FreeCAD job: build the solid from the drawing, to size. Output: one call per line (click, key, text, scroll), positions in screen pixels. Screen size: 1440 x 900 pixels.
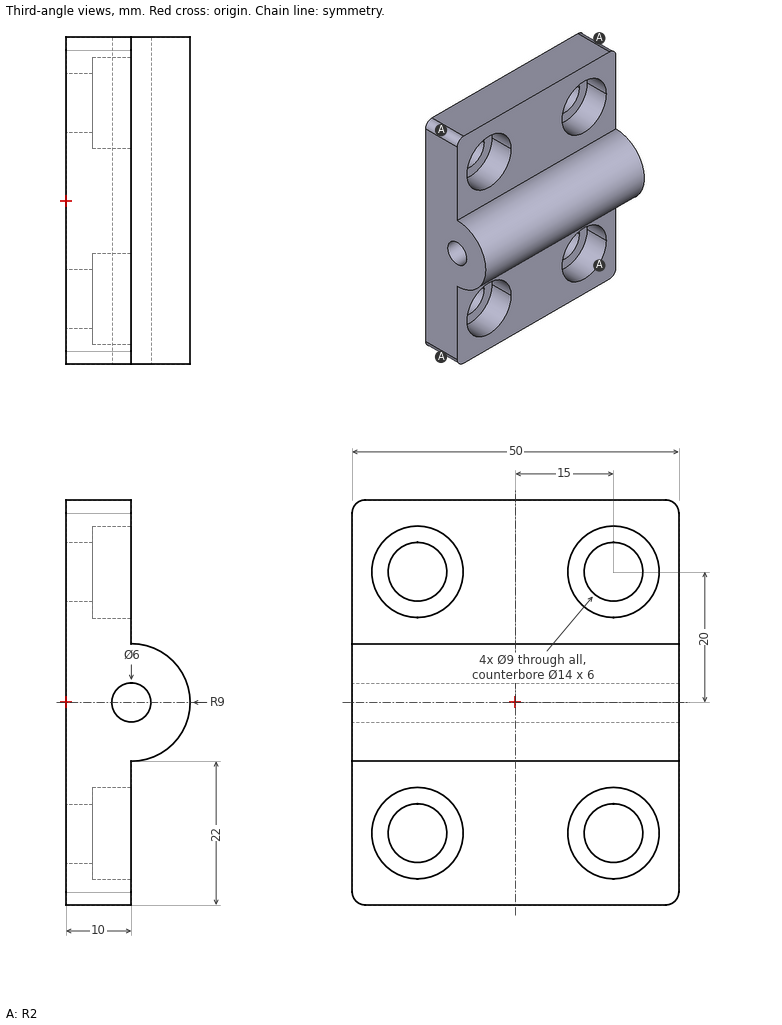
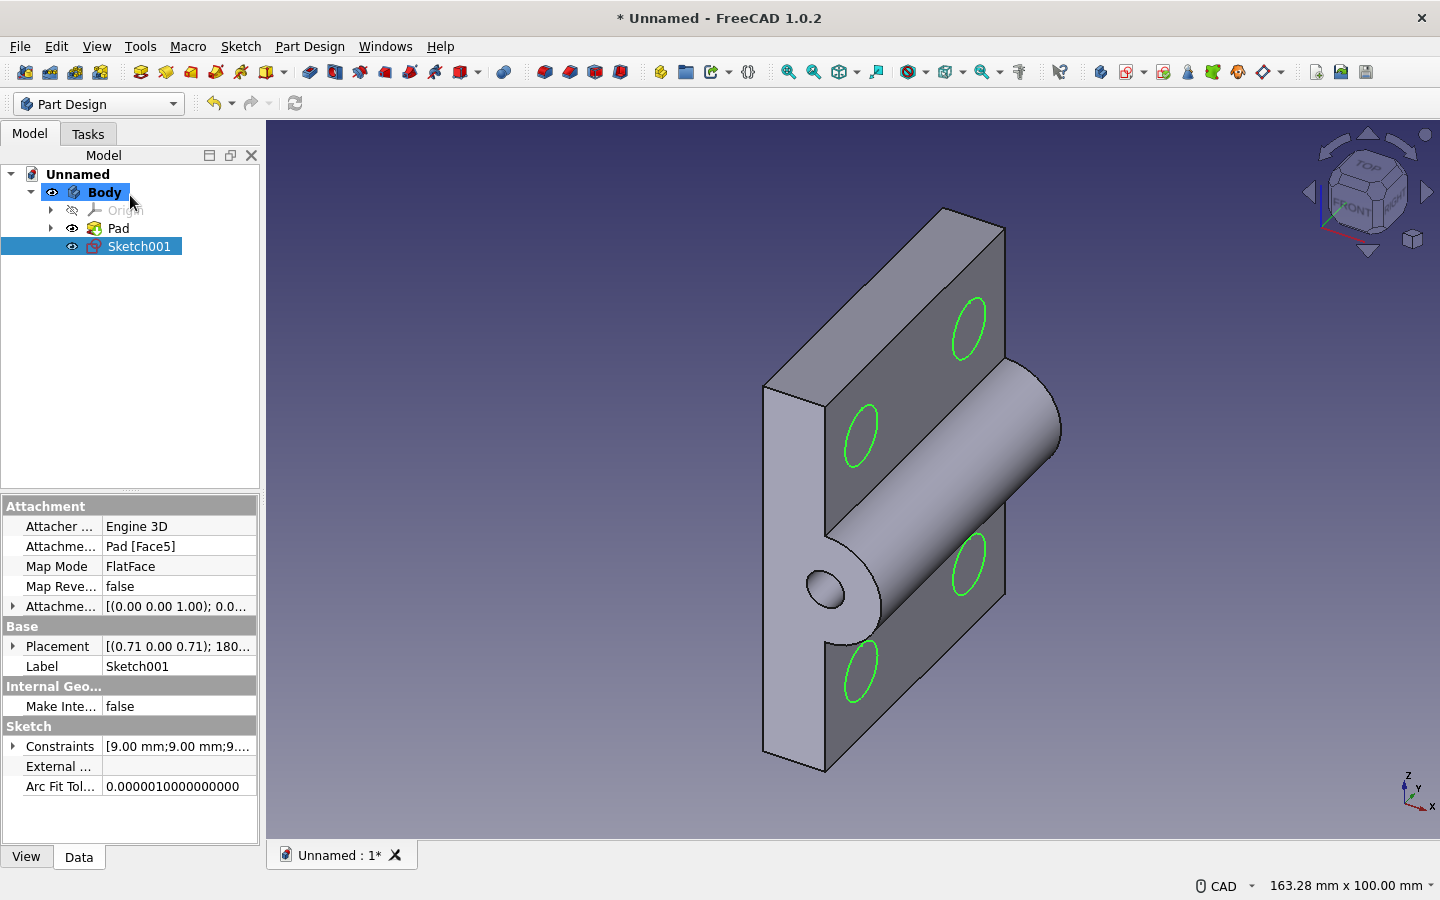
click(335, 72)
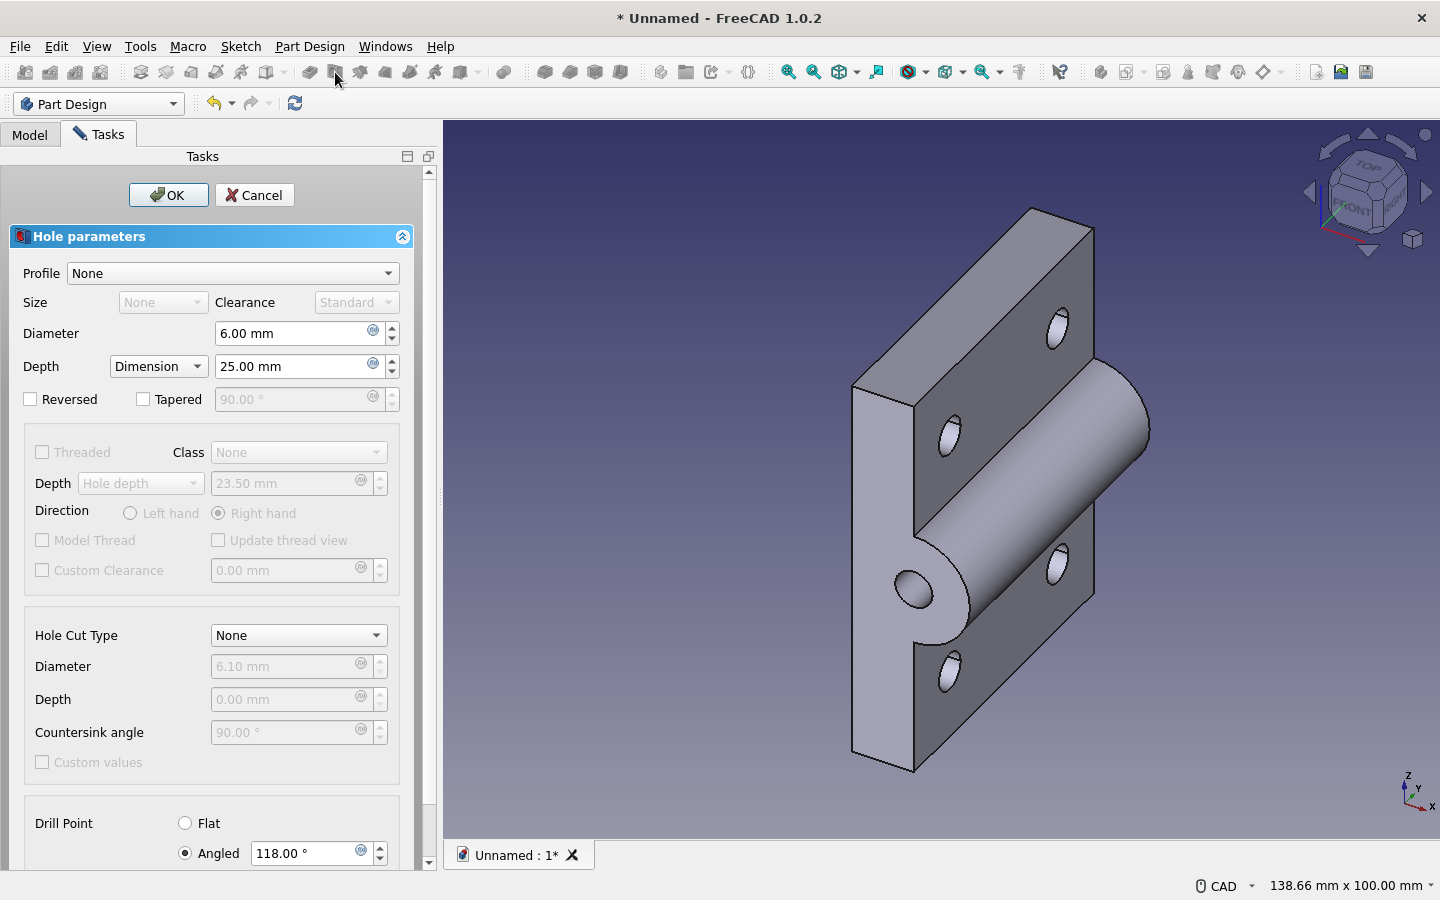
triple_click(300, 334)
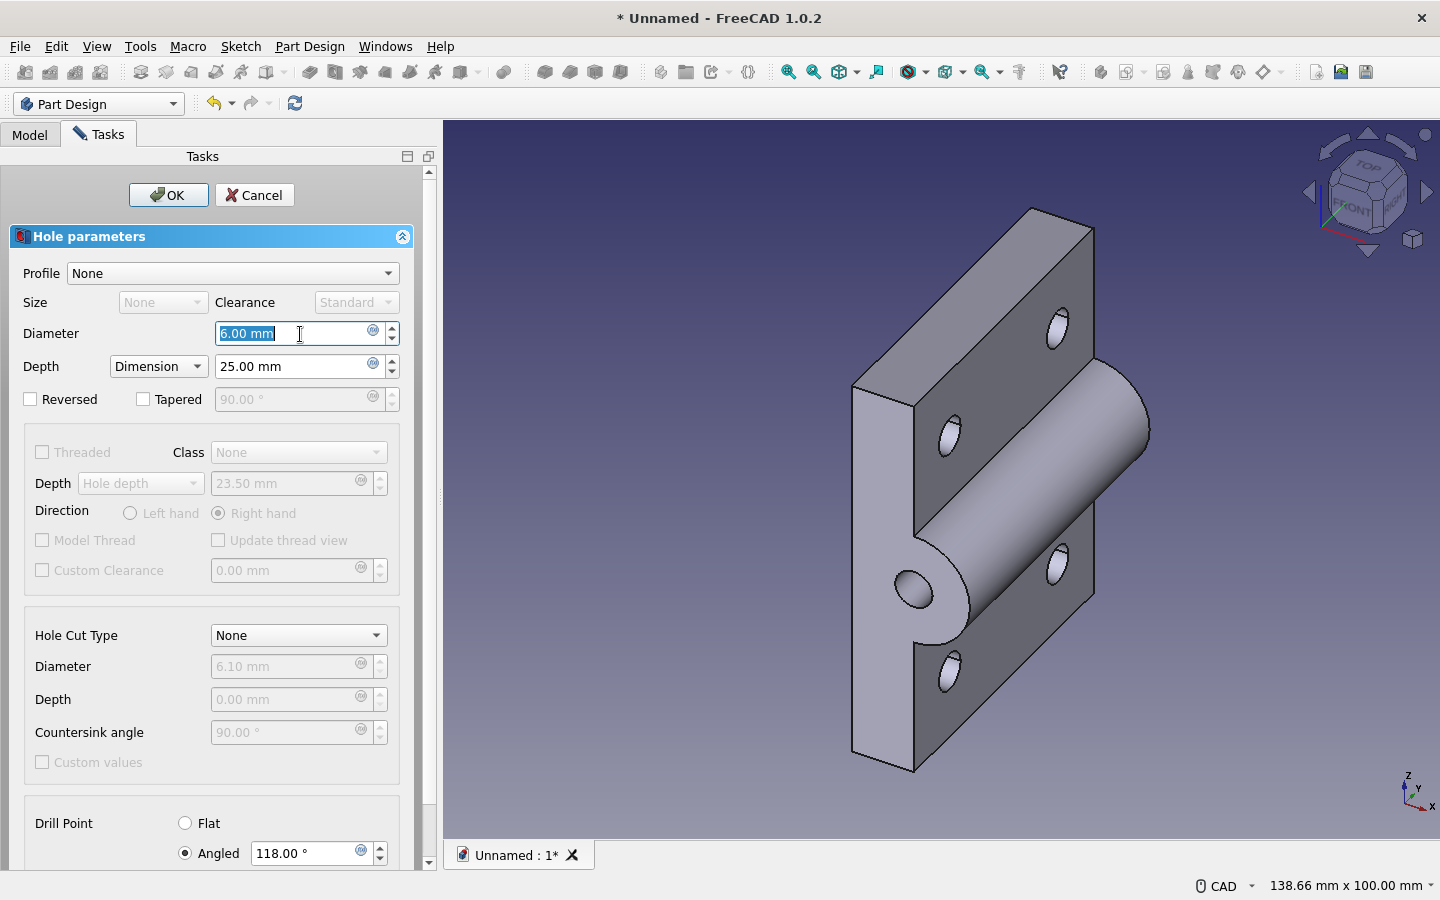
text(9)
key(Tab)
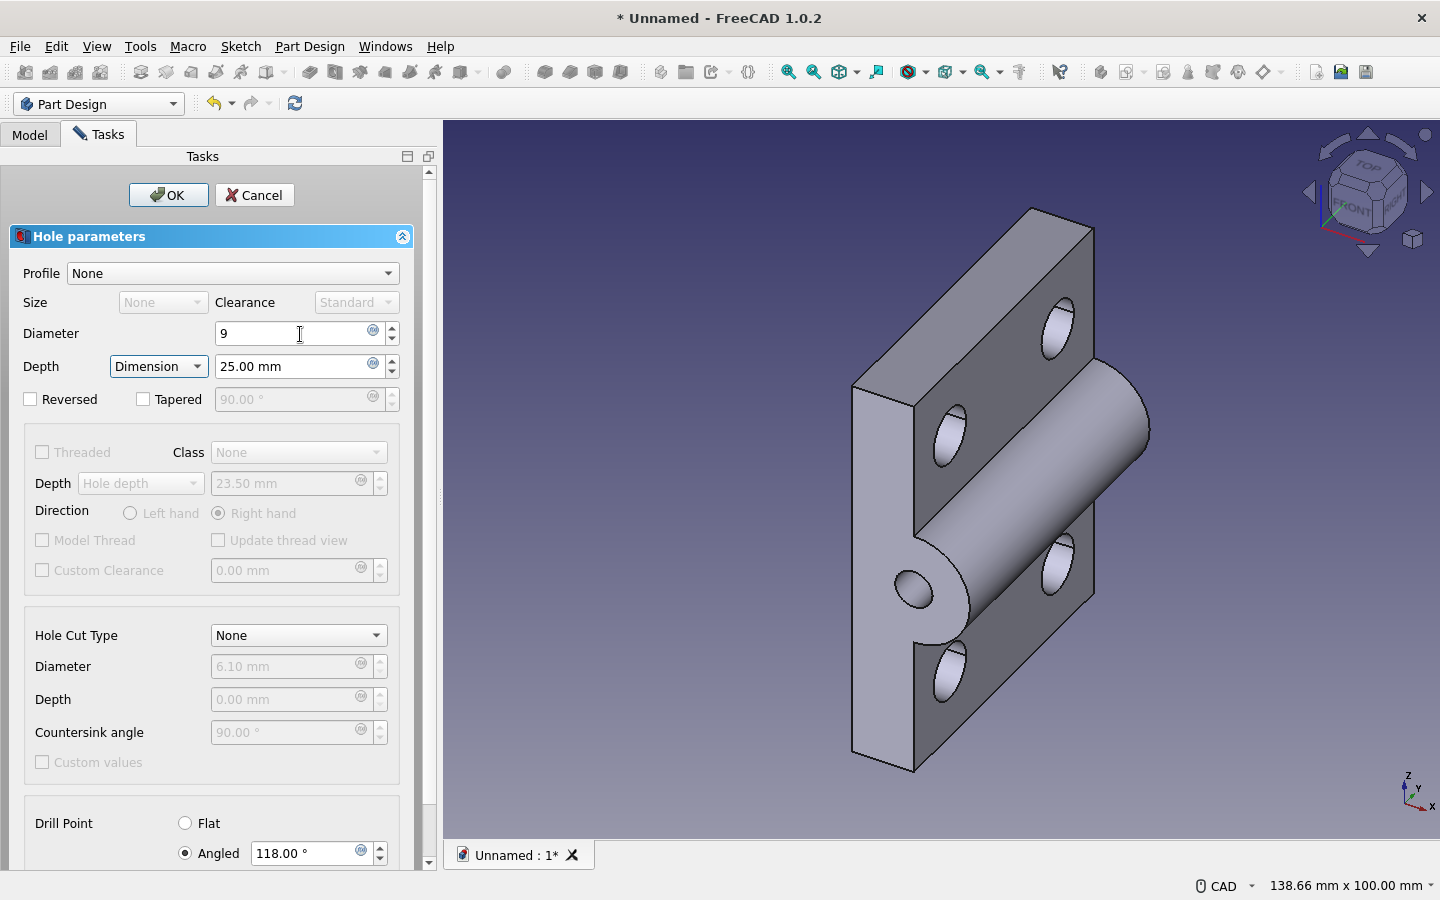
click(160, 366)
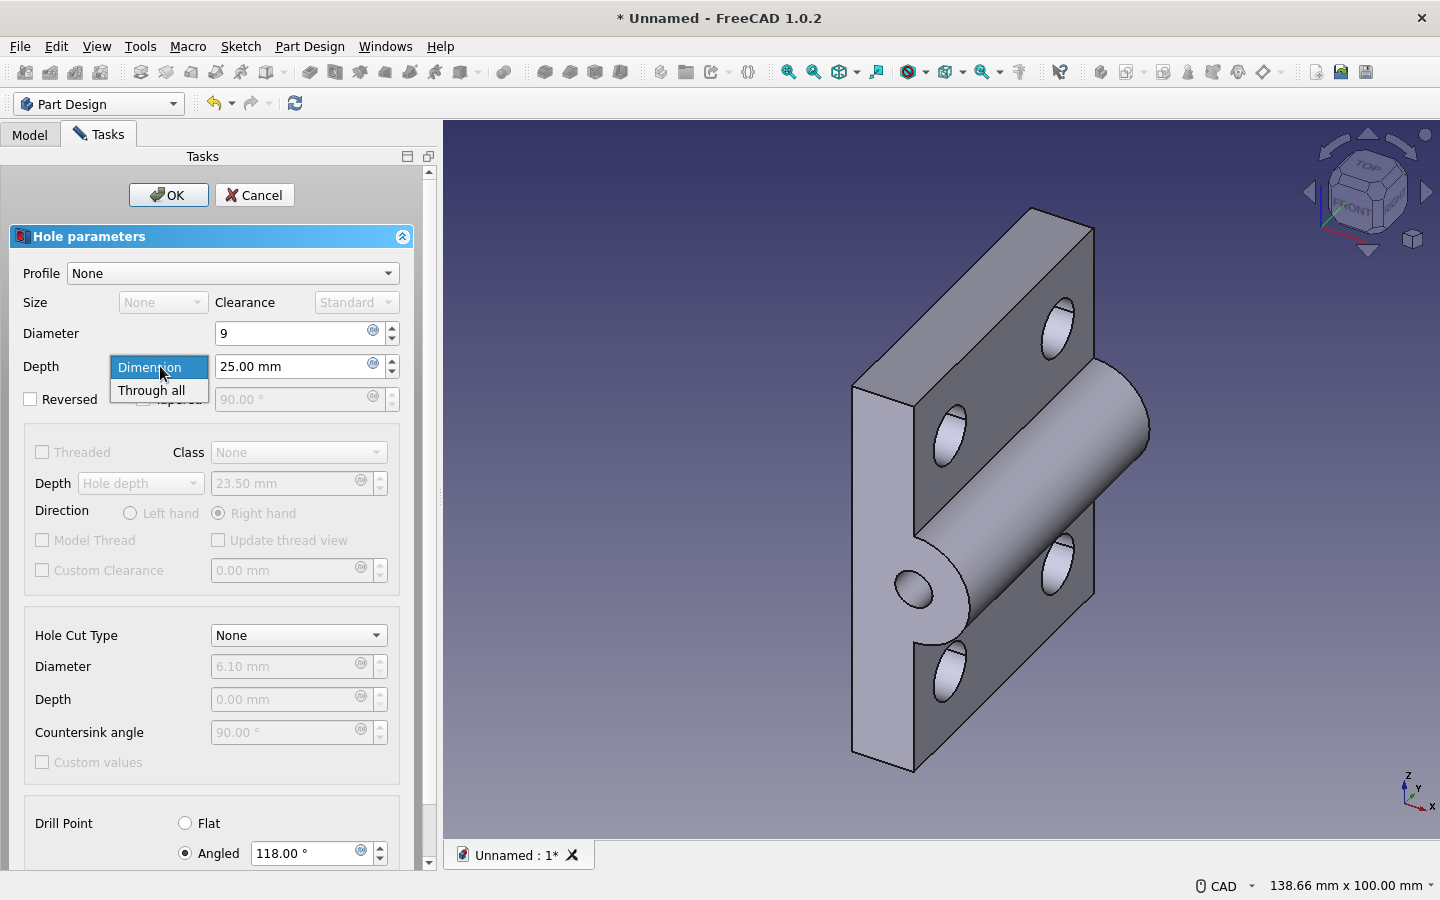
click(158, 390)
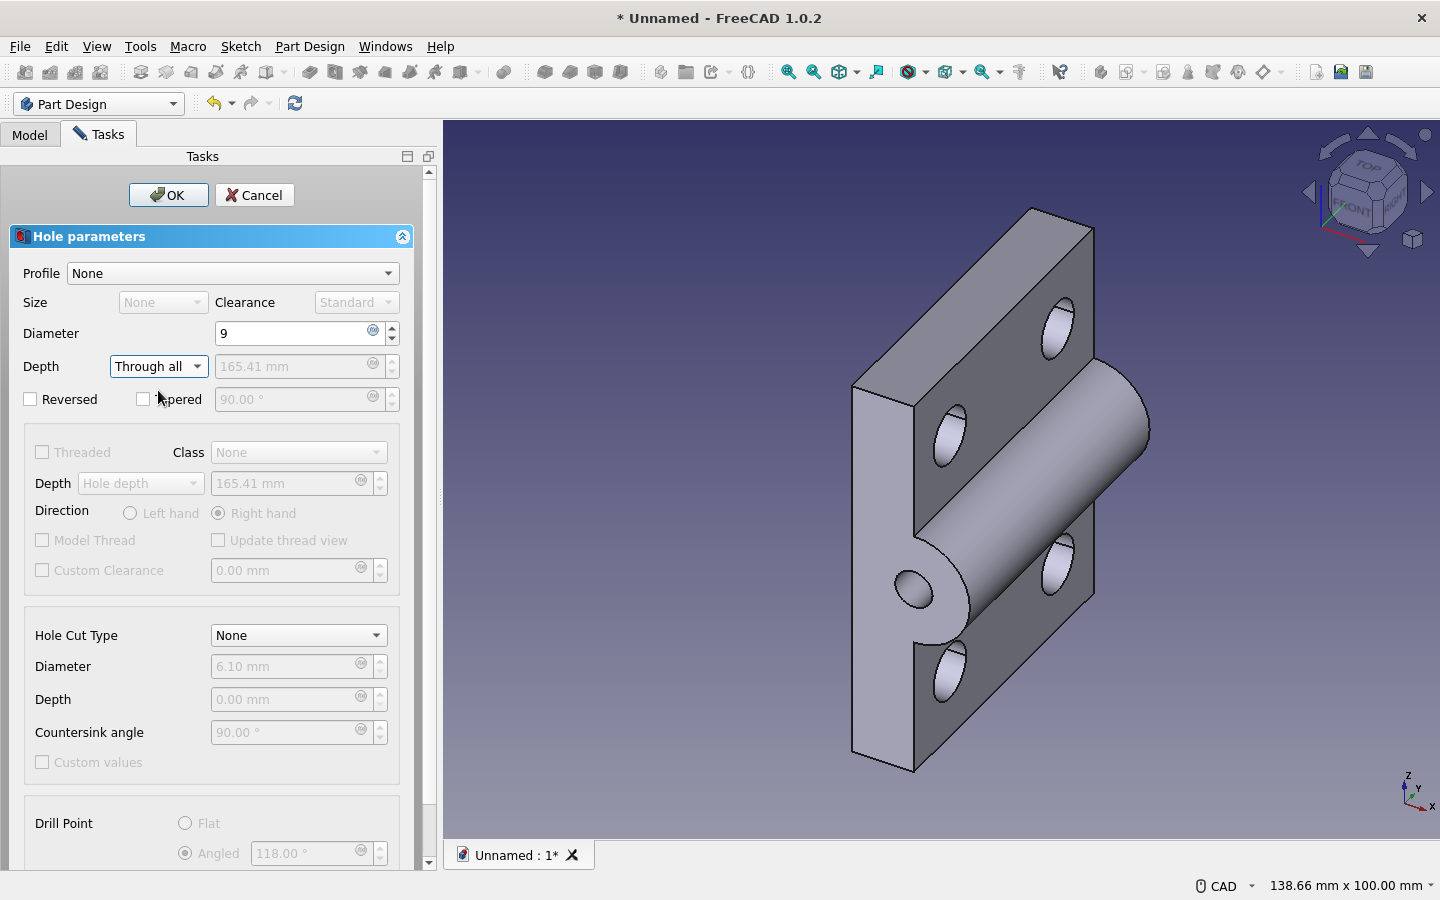
click(300, 636)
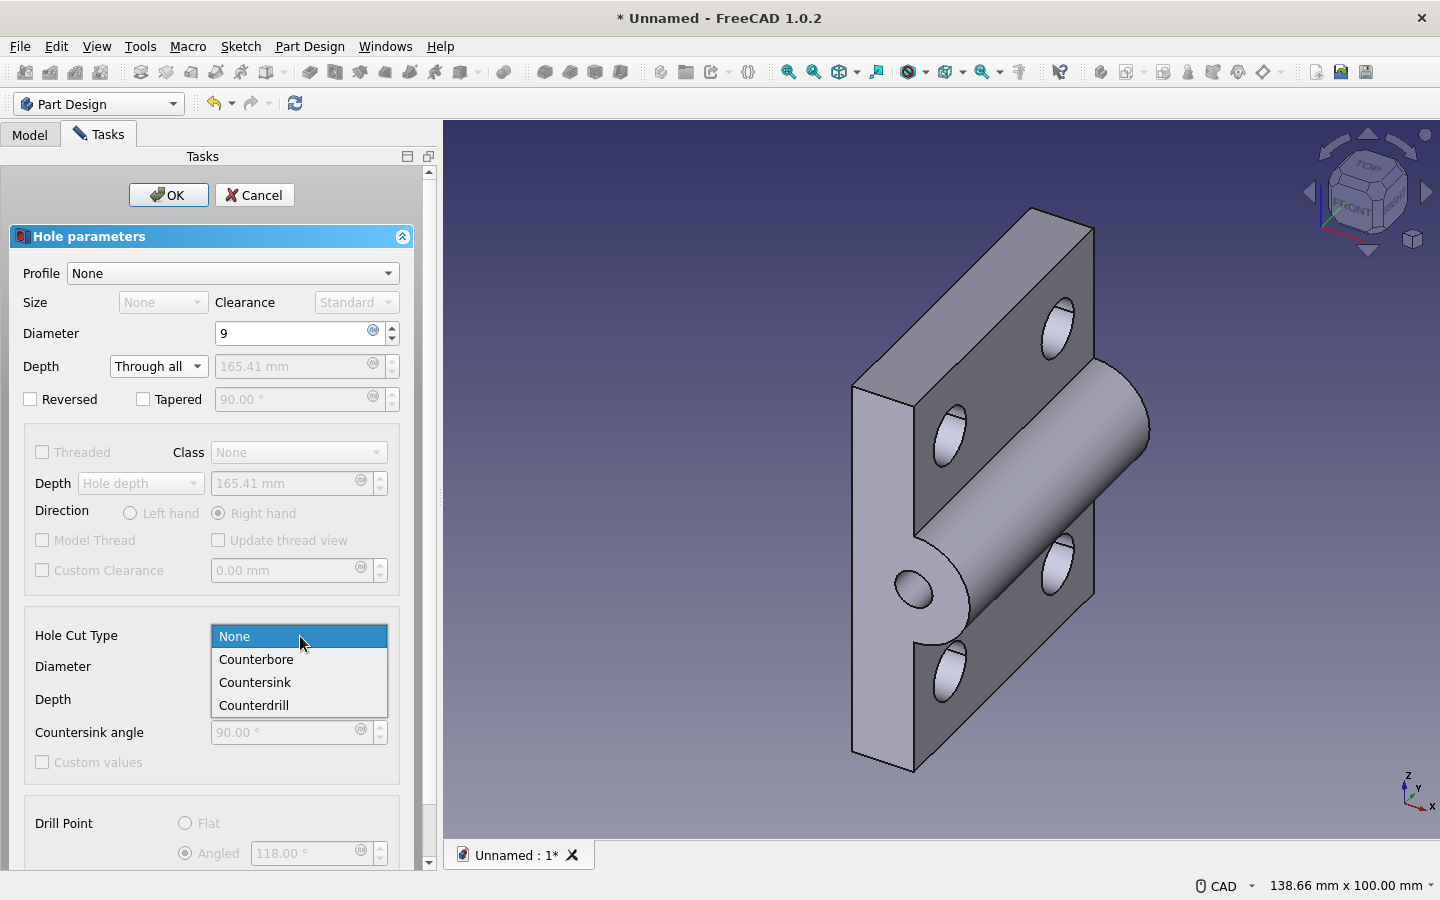
click(298, 660)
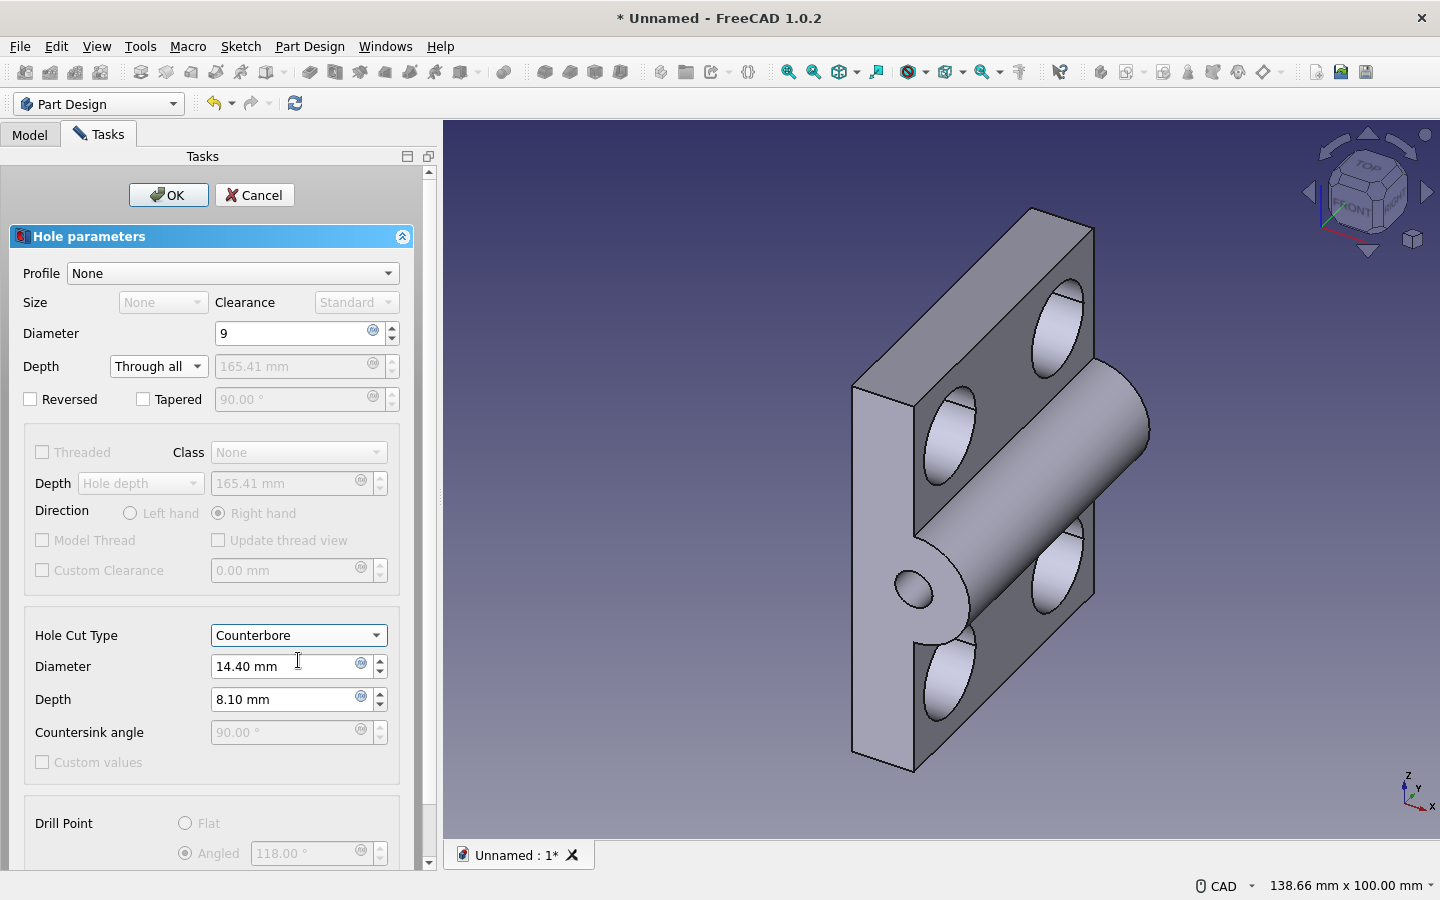
triple_click(292, 666)